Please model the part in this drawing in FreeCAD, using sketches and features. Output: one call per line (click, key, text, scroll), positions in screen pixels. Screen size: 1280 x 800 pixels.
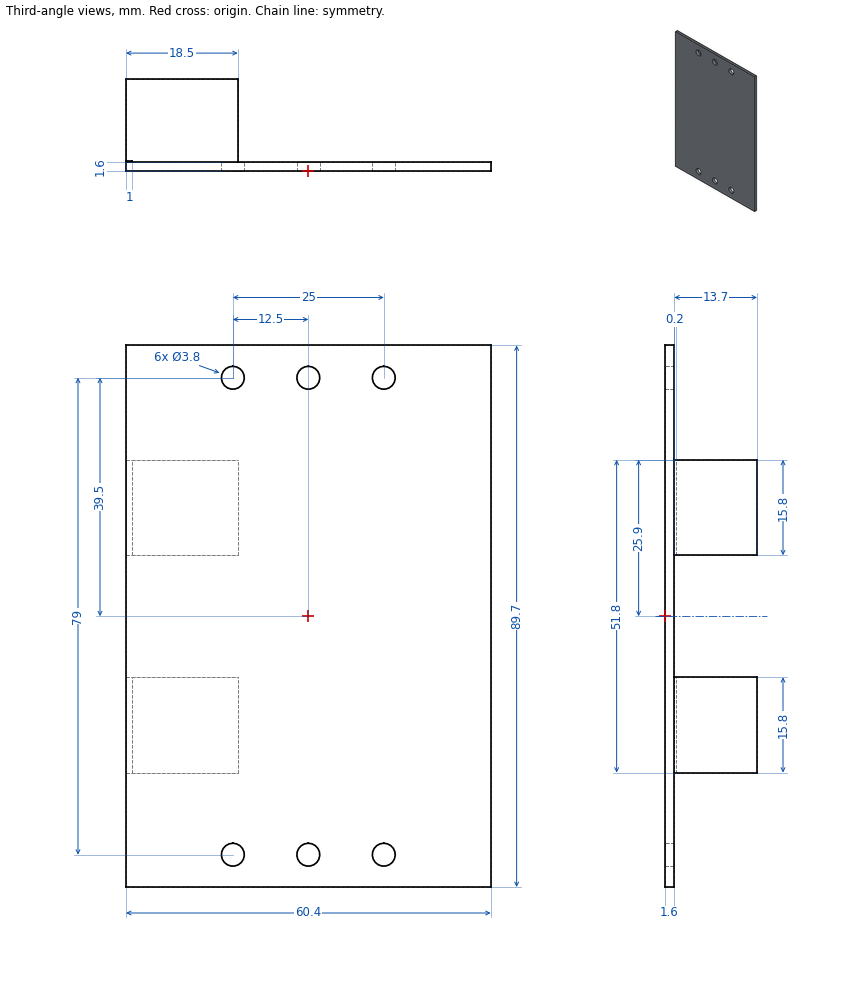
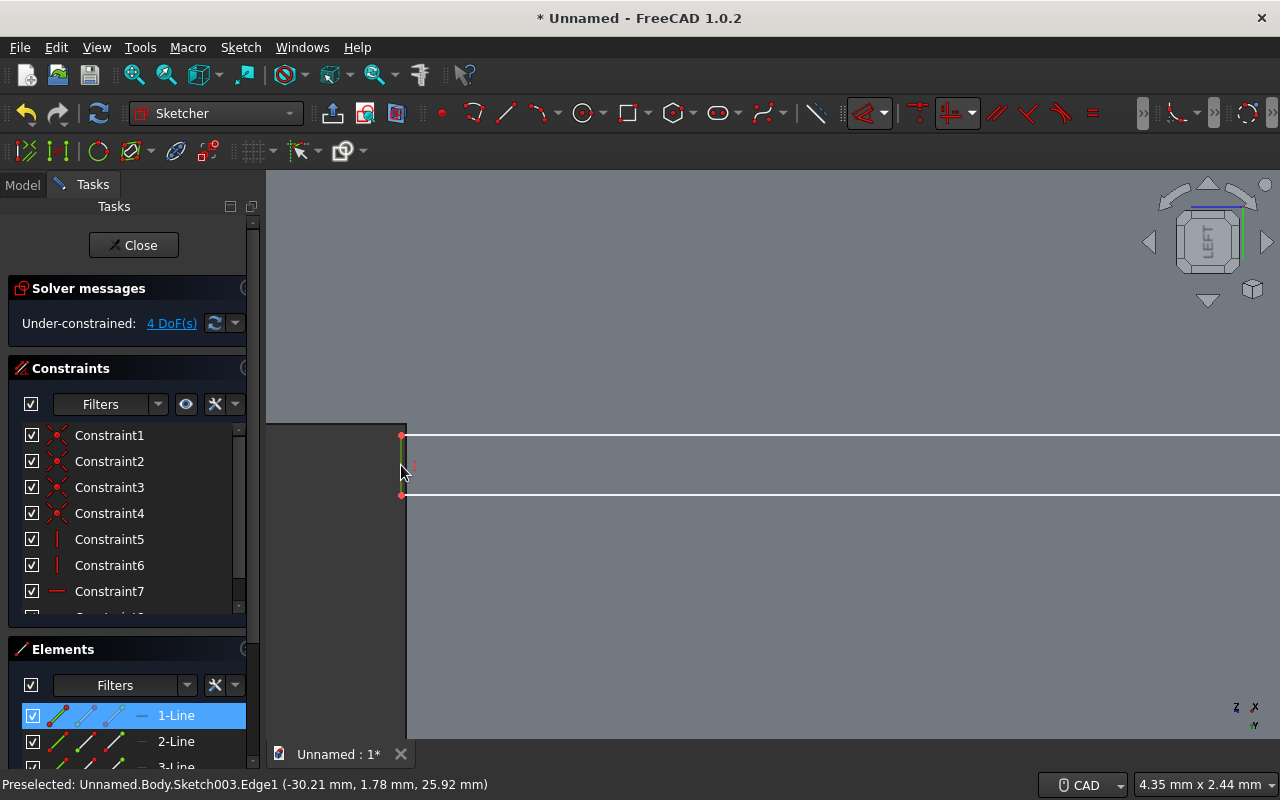
click(886, 114)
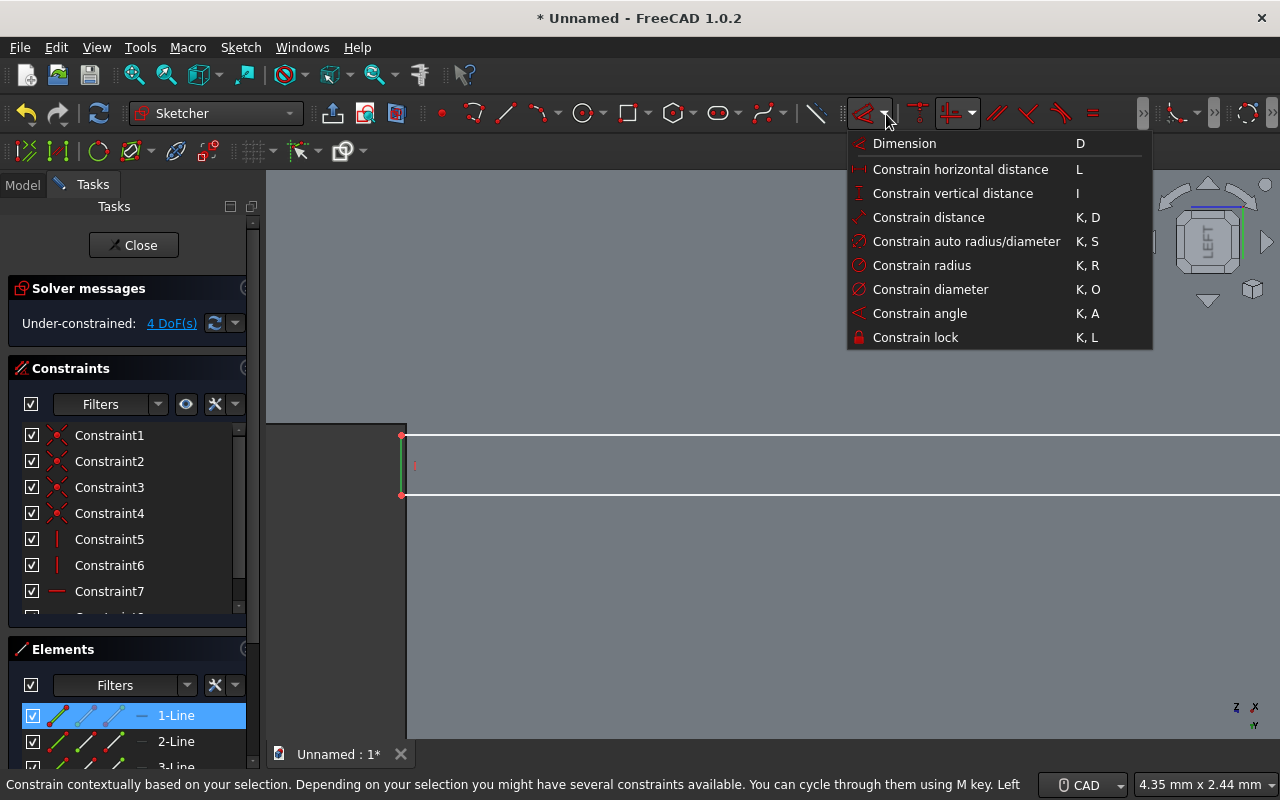
click(1000, 193)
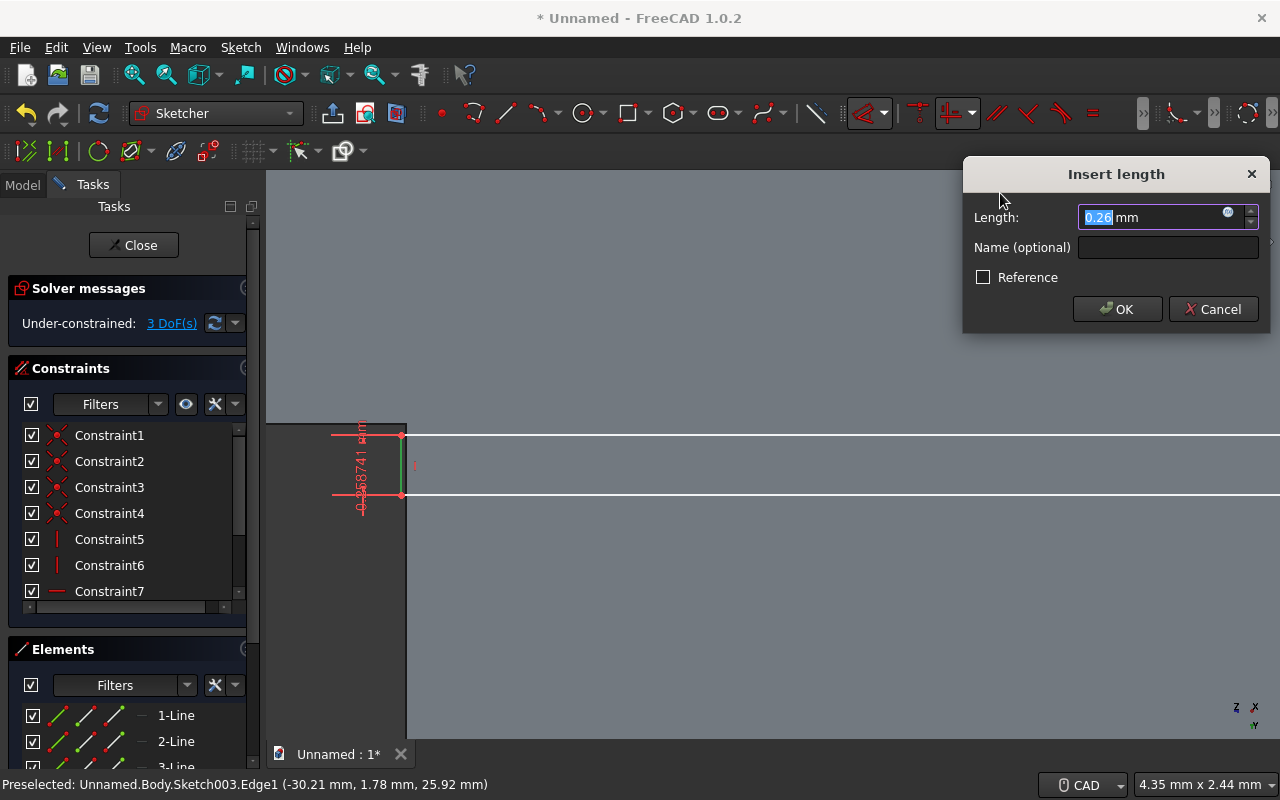
text(0.2)
key(Return)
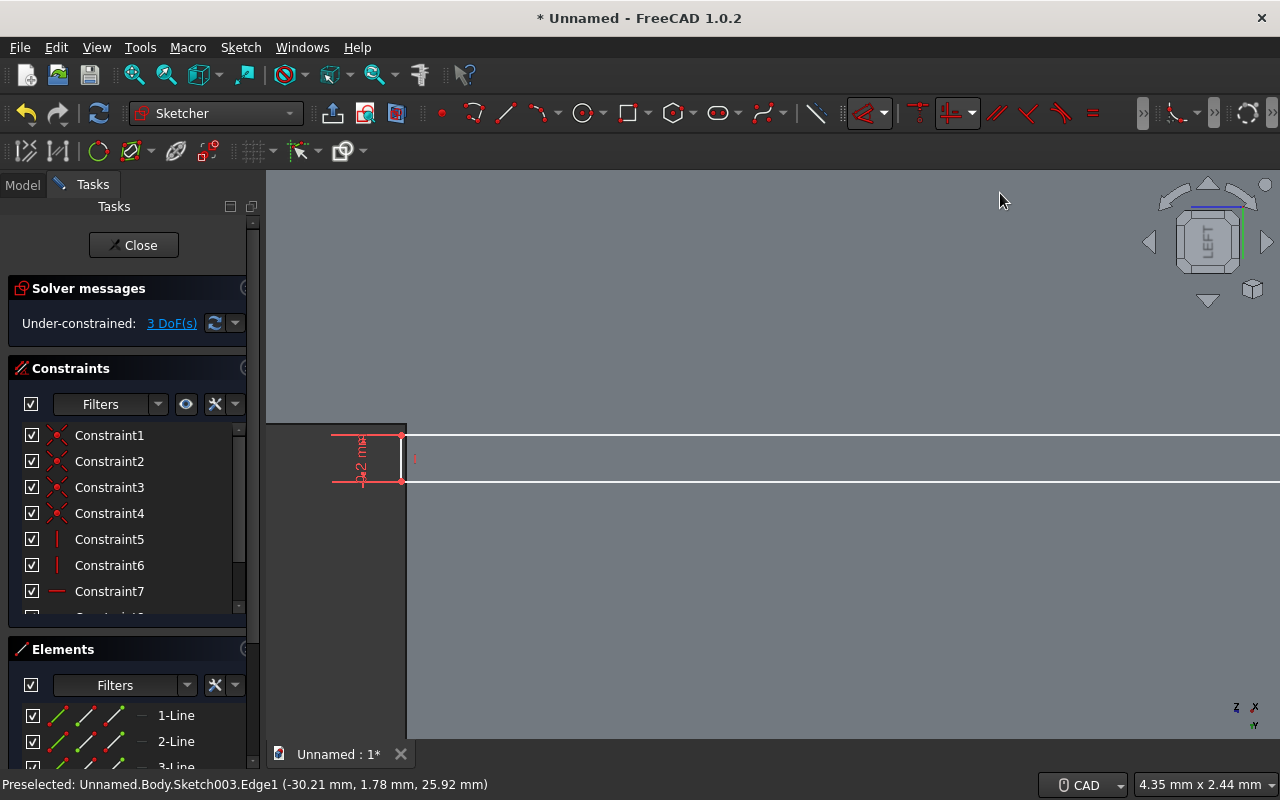
scroll(404, 465, down, 15)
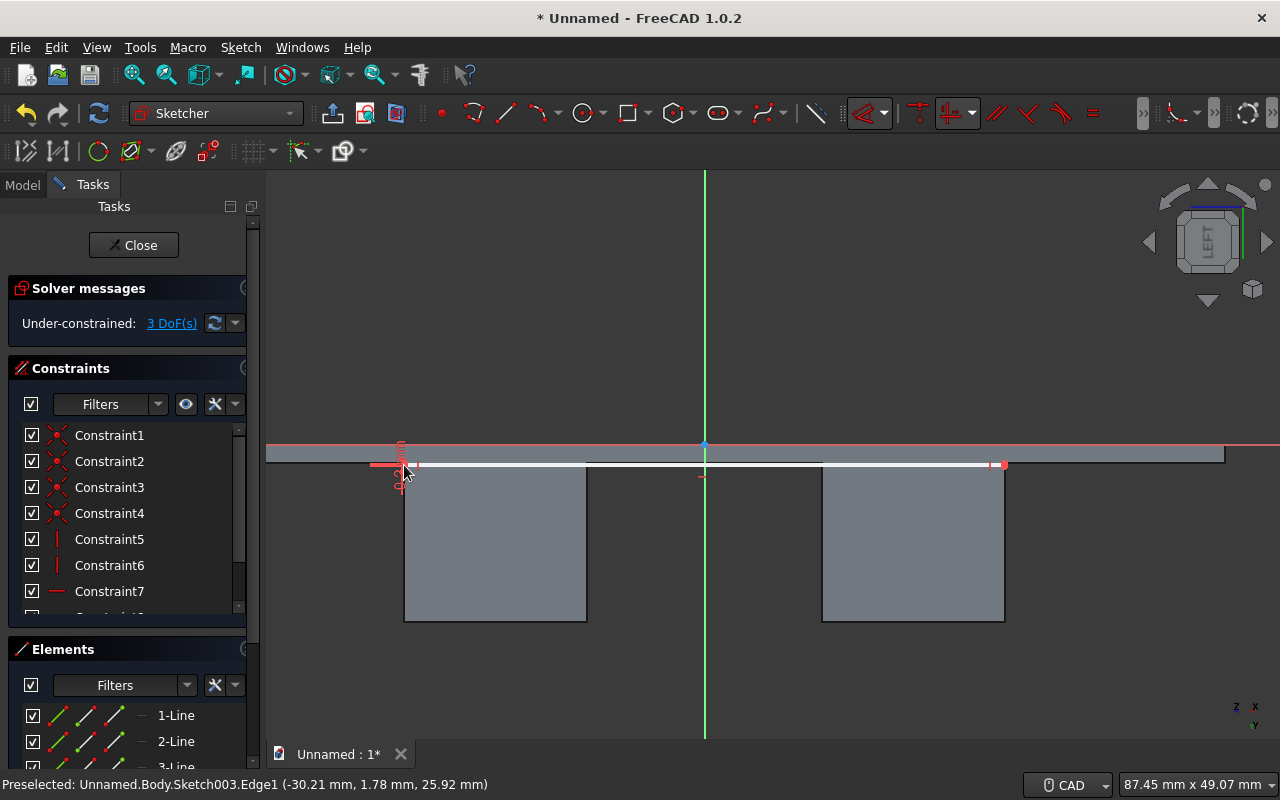
scroll(584, 466, up, 9)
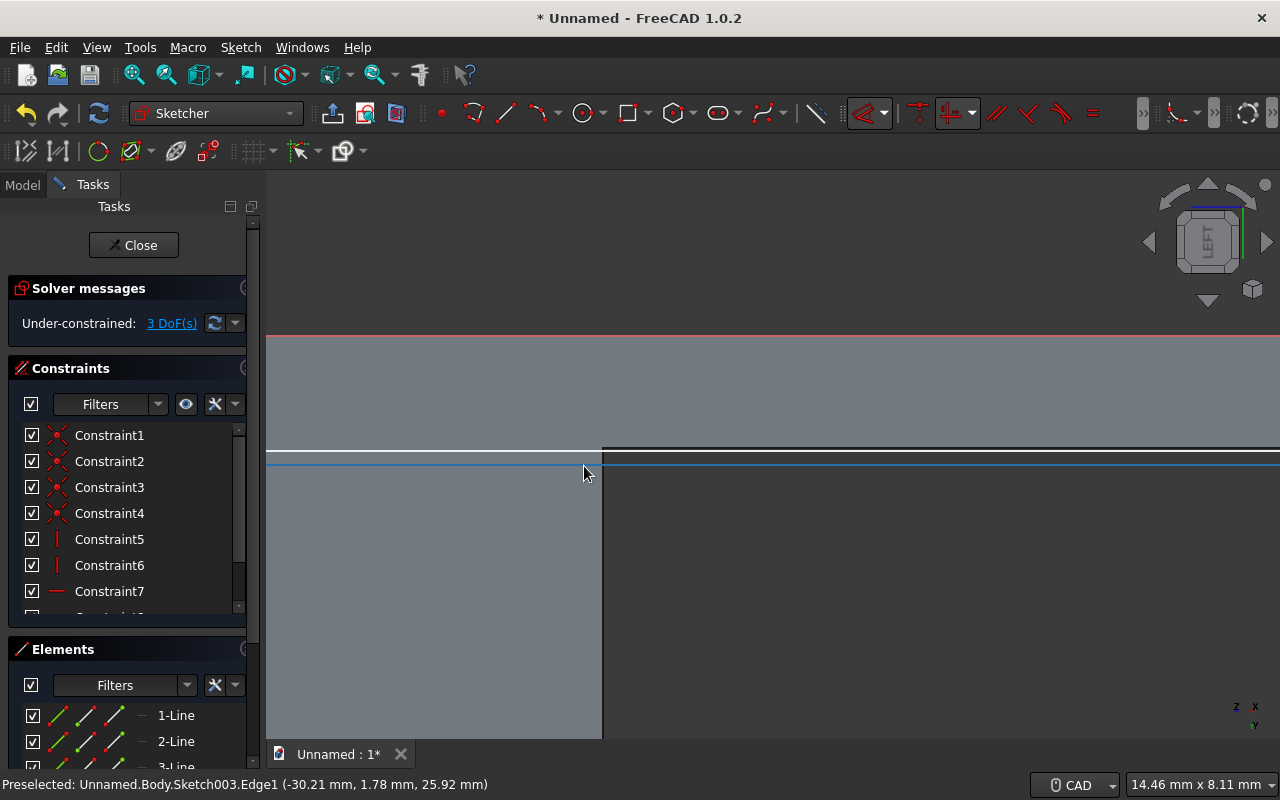
click(584, 465)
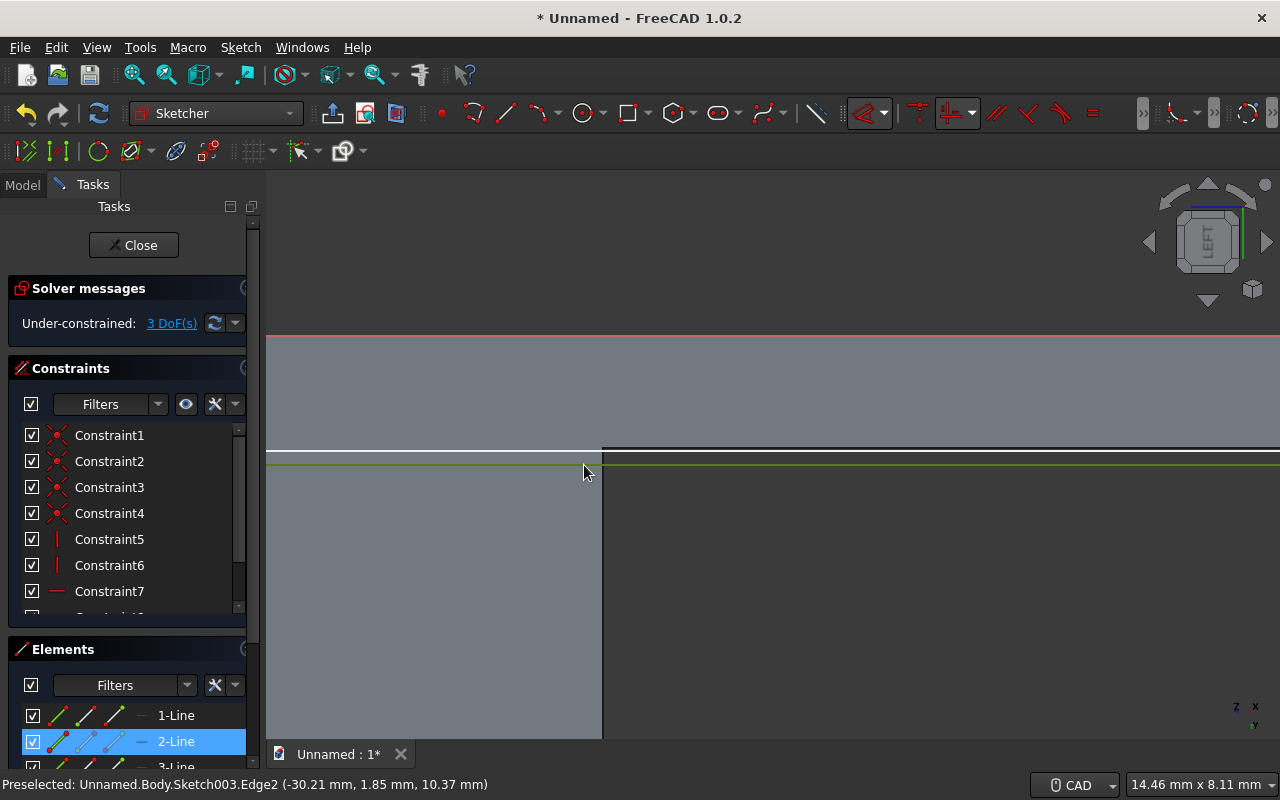
key(l)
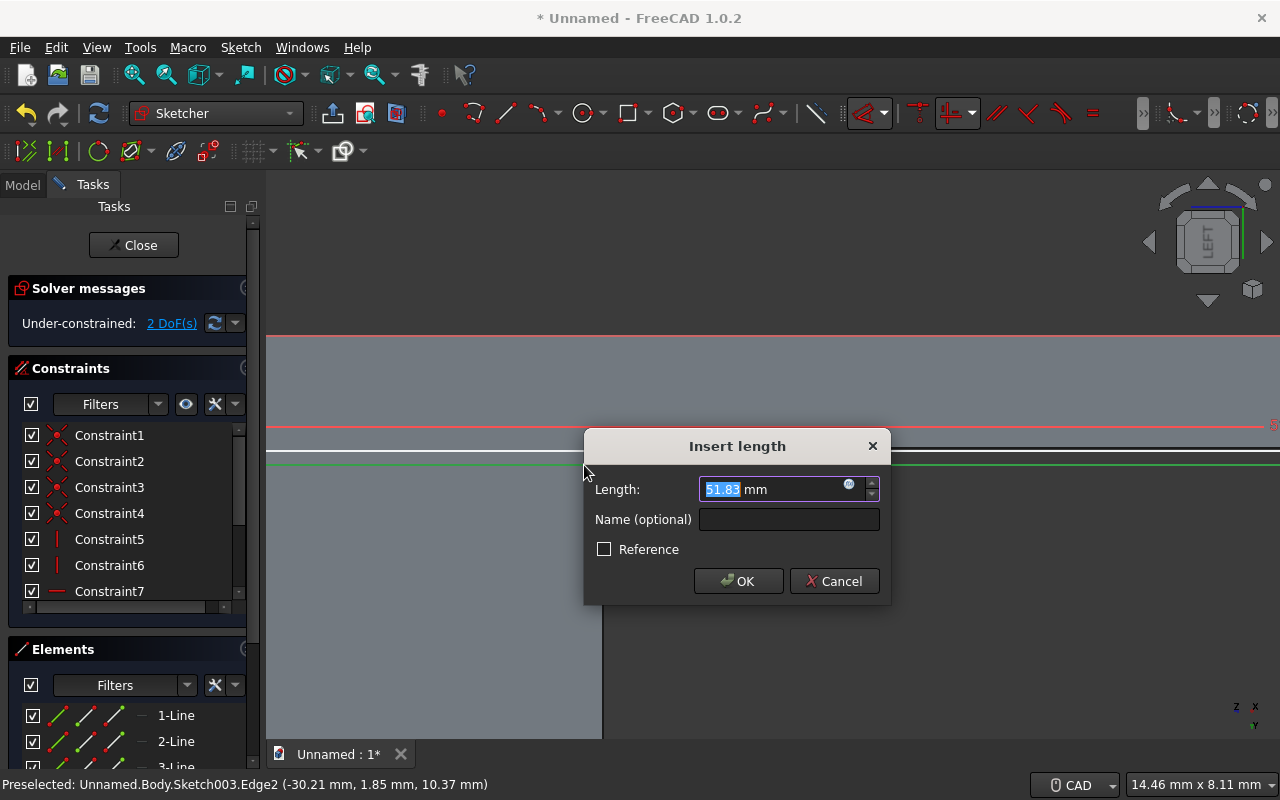
text(51.8)
key(Return)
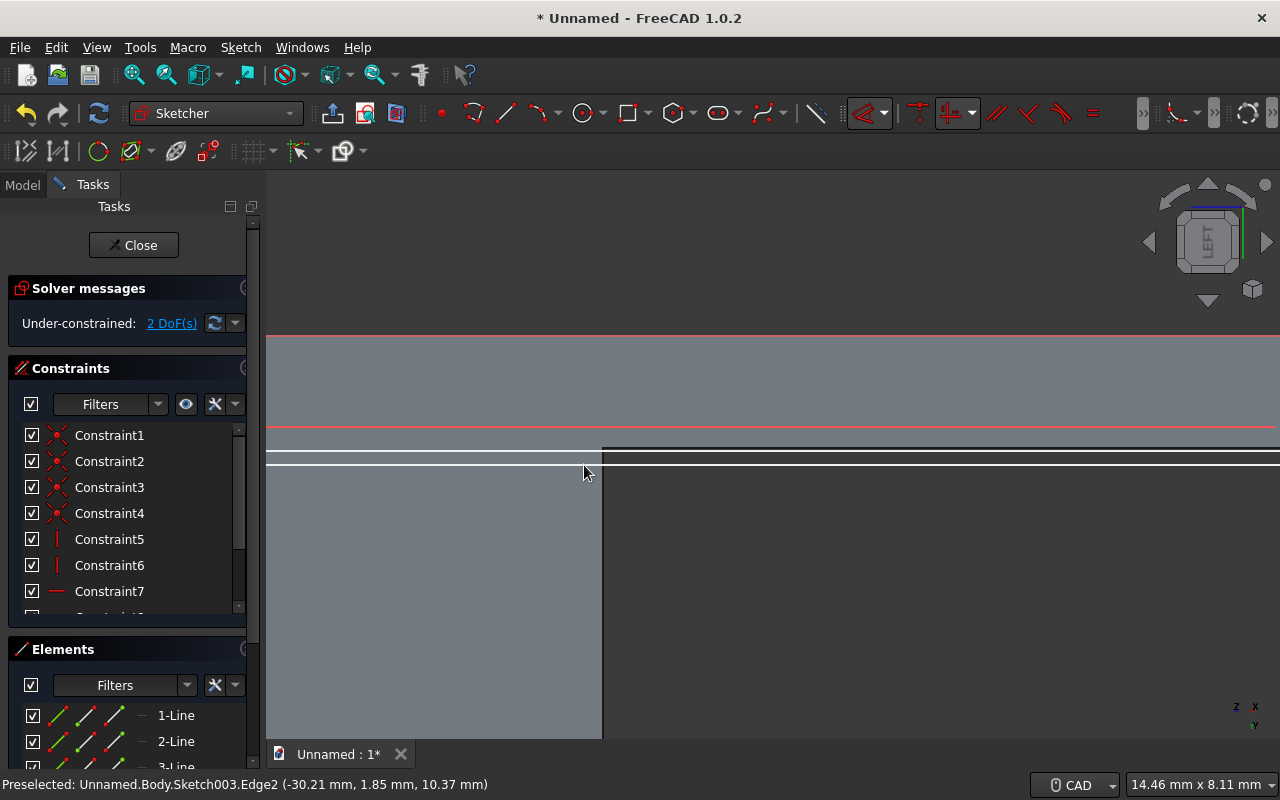
scroll(584, 466, down, 9)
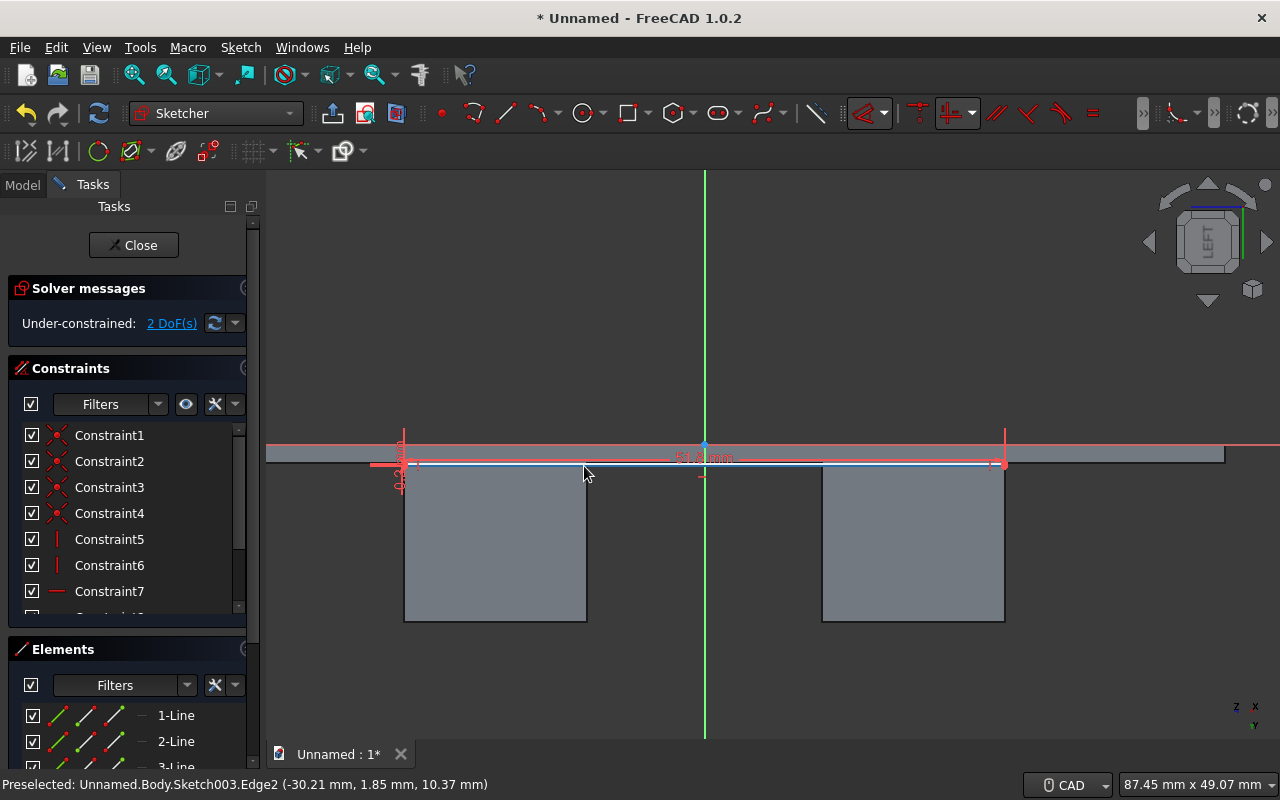
scroll(404, 464, up, 9)